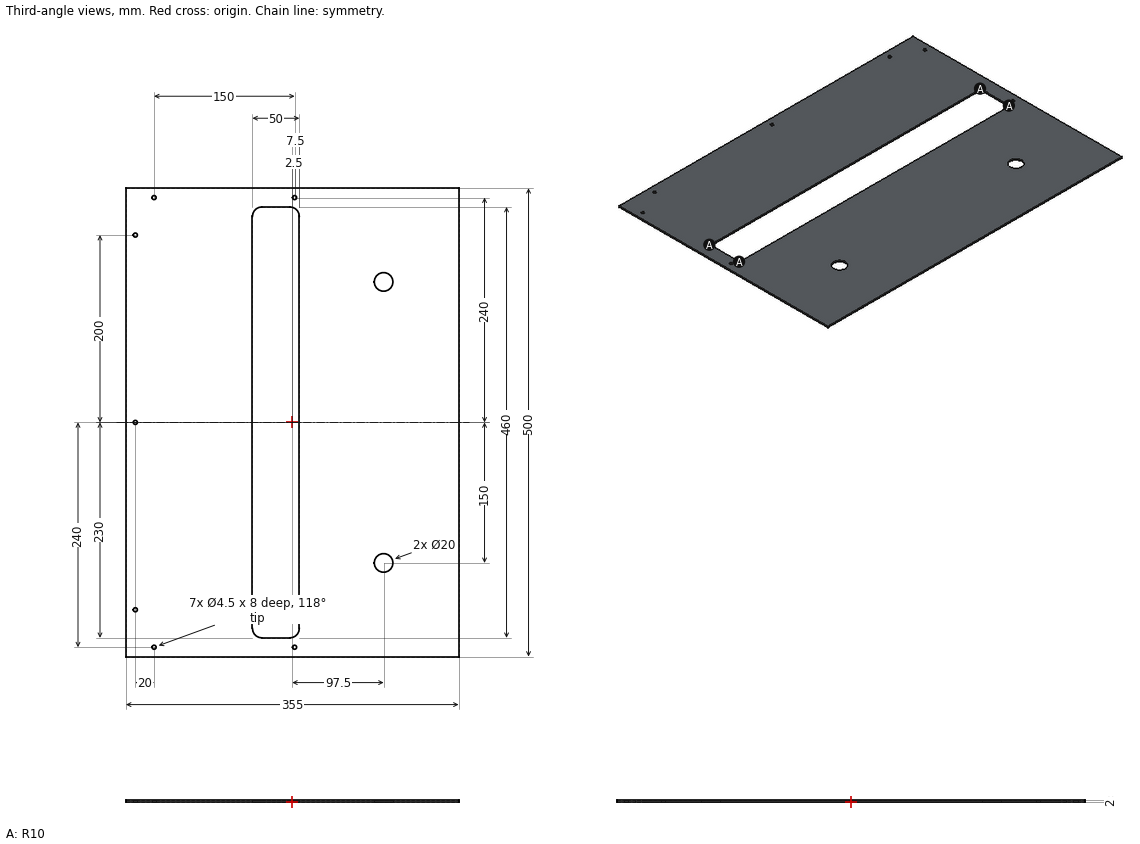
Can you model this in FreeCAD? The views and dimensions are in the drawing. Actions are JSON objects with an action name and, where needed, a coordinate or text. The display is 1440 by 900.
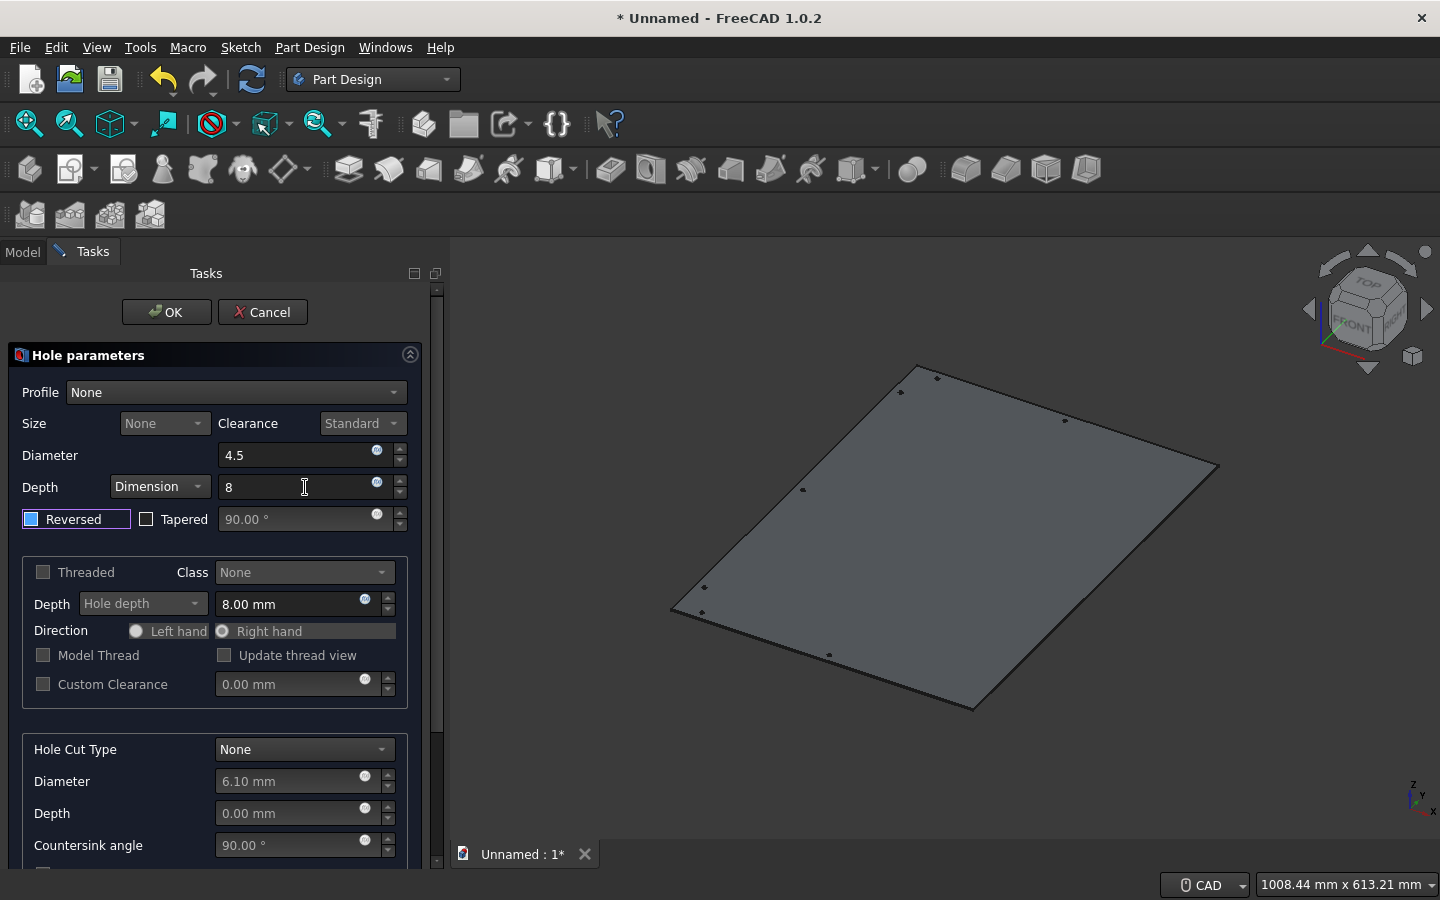
{"action": "left_click", "coordinate": [167, 312]}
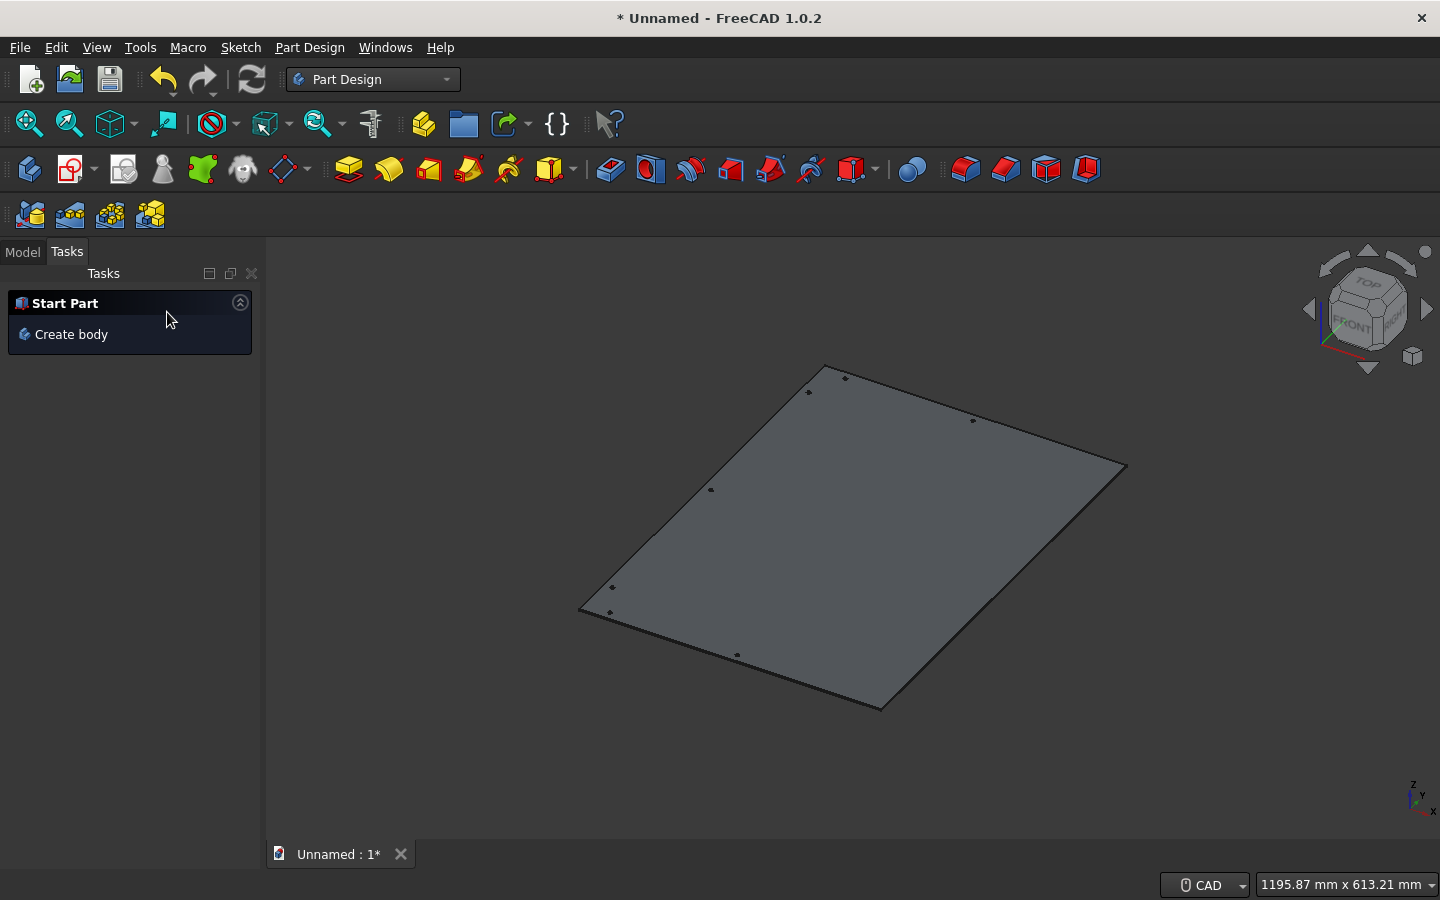
{"action": "key", "text": "5"}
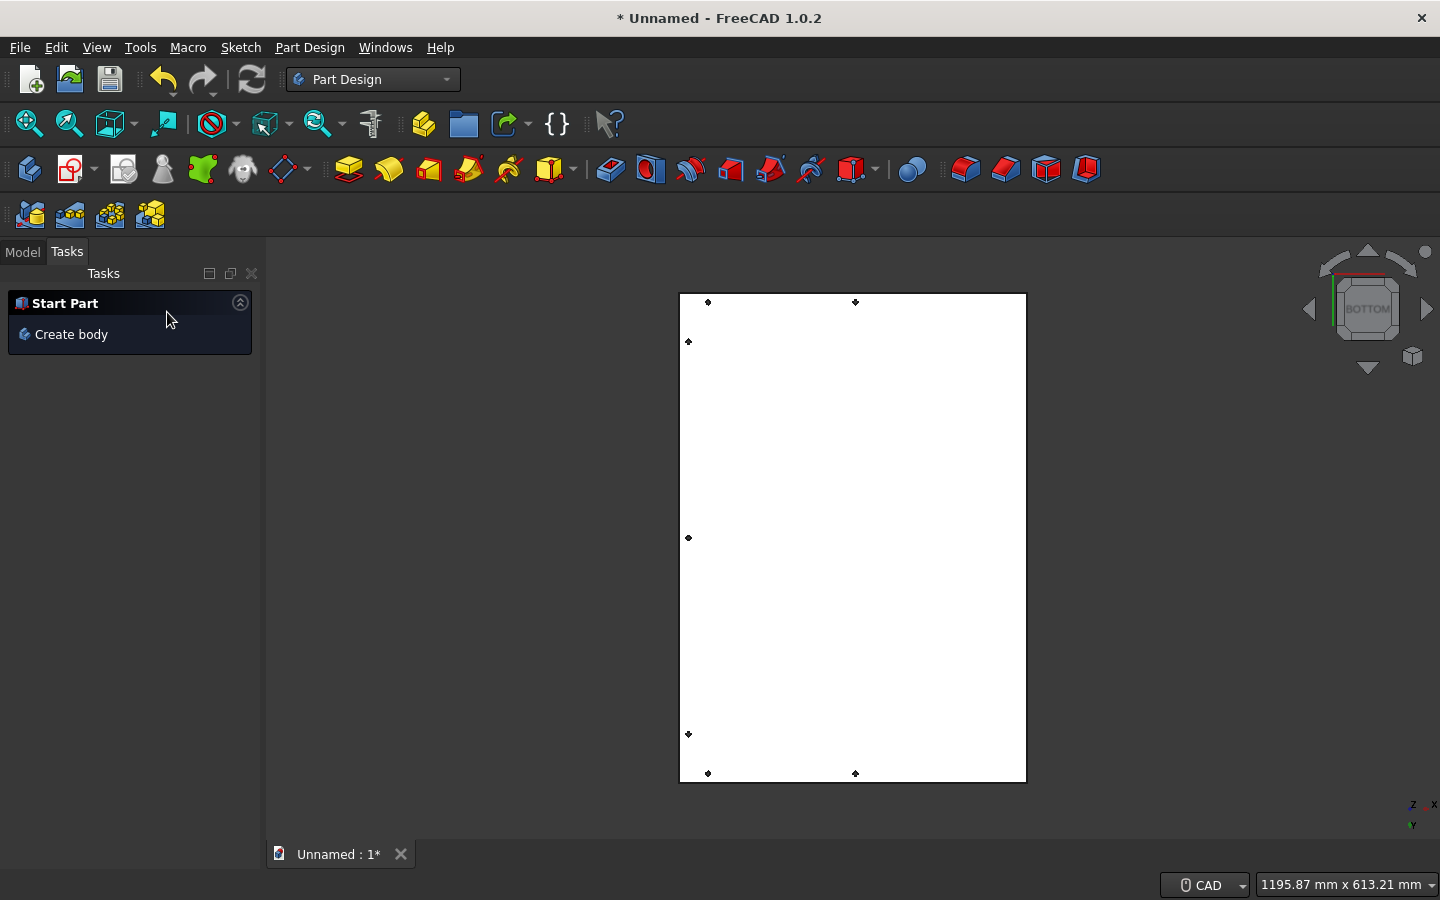
{"action": "left_click", "coordinate": [853, 467]}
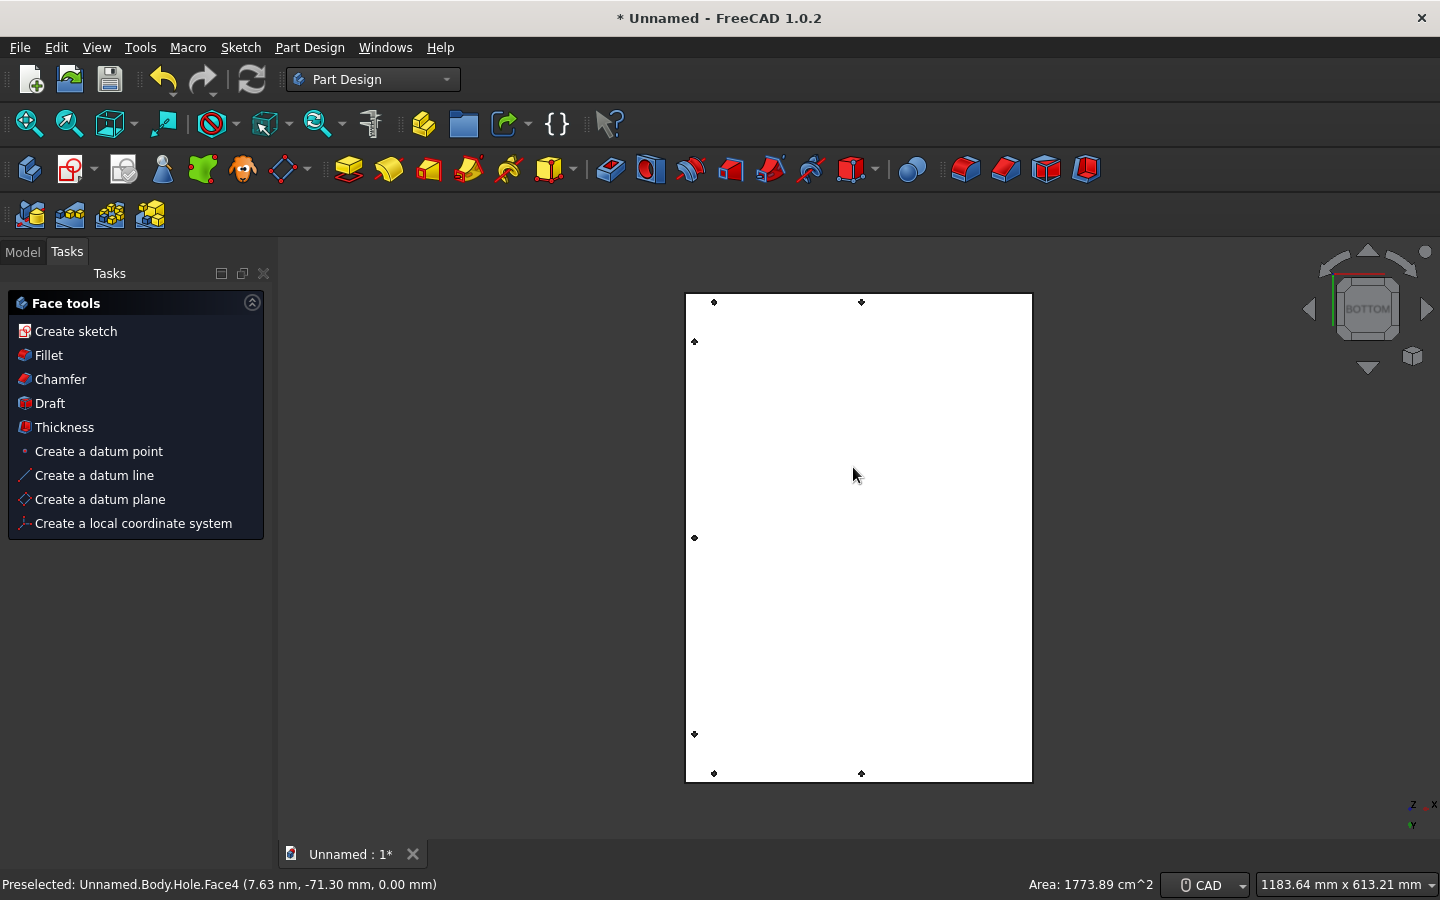
{"action": "left_click", "coordinate": [70, 170]}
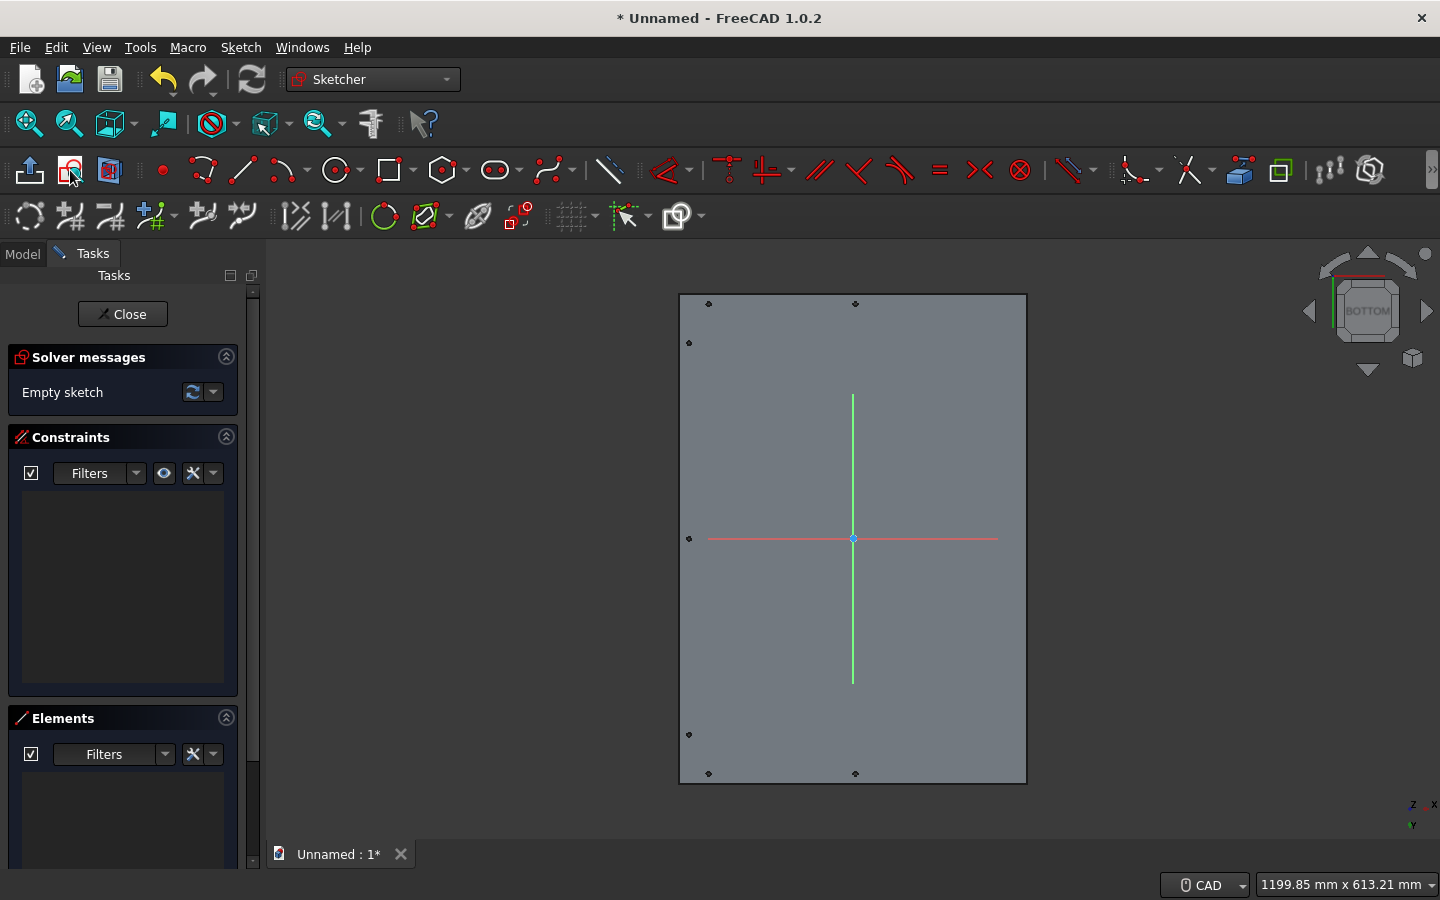
{"action": "left_click", "coordinate": [390, 170]}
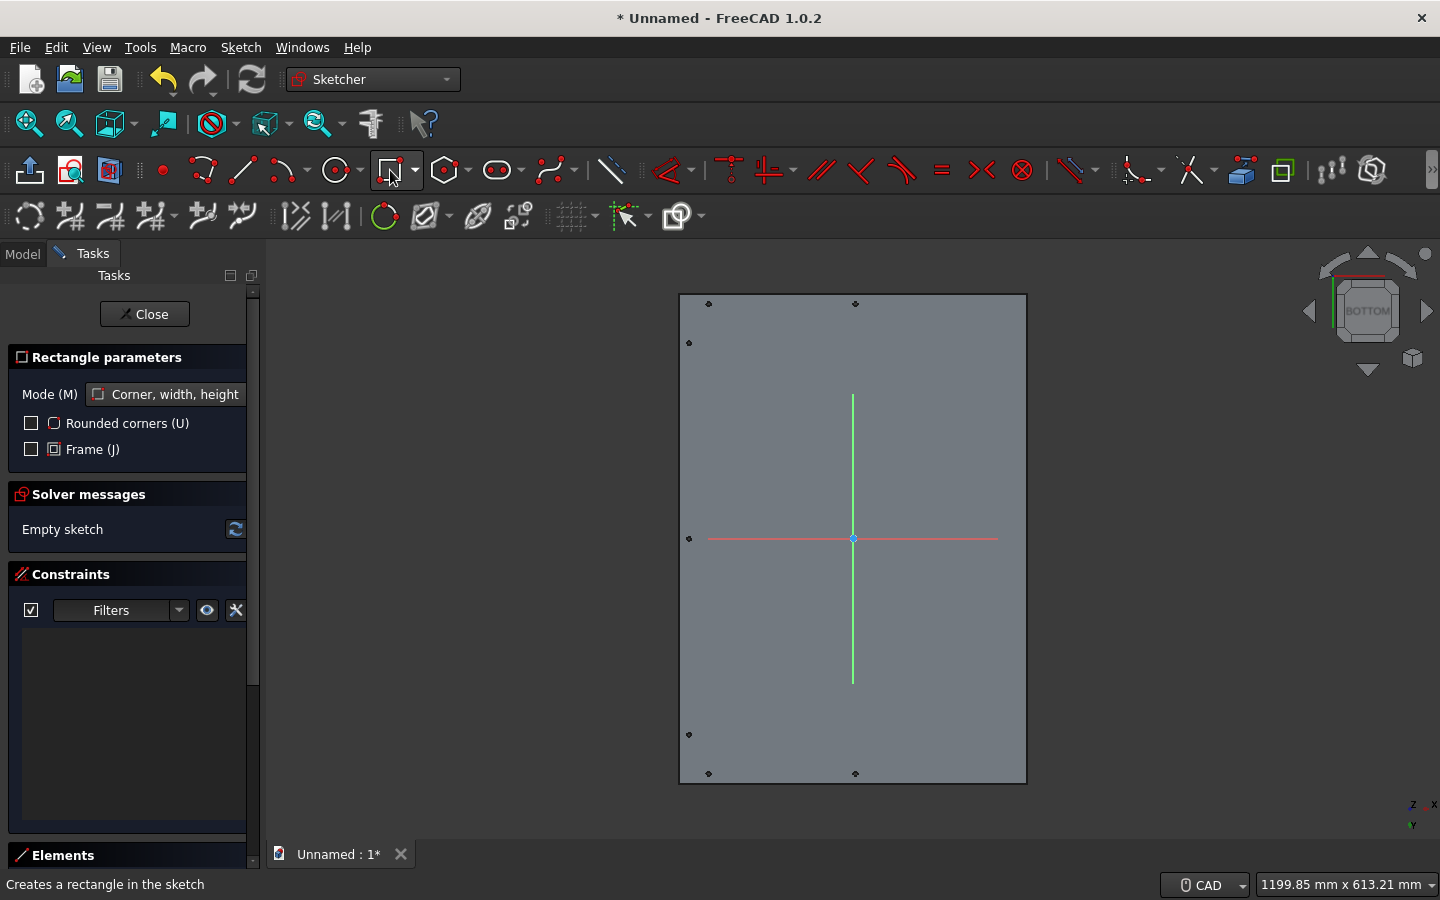
{"action": "left_click", "coordinate": [811, 314]}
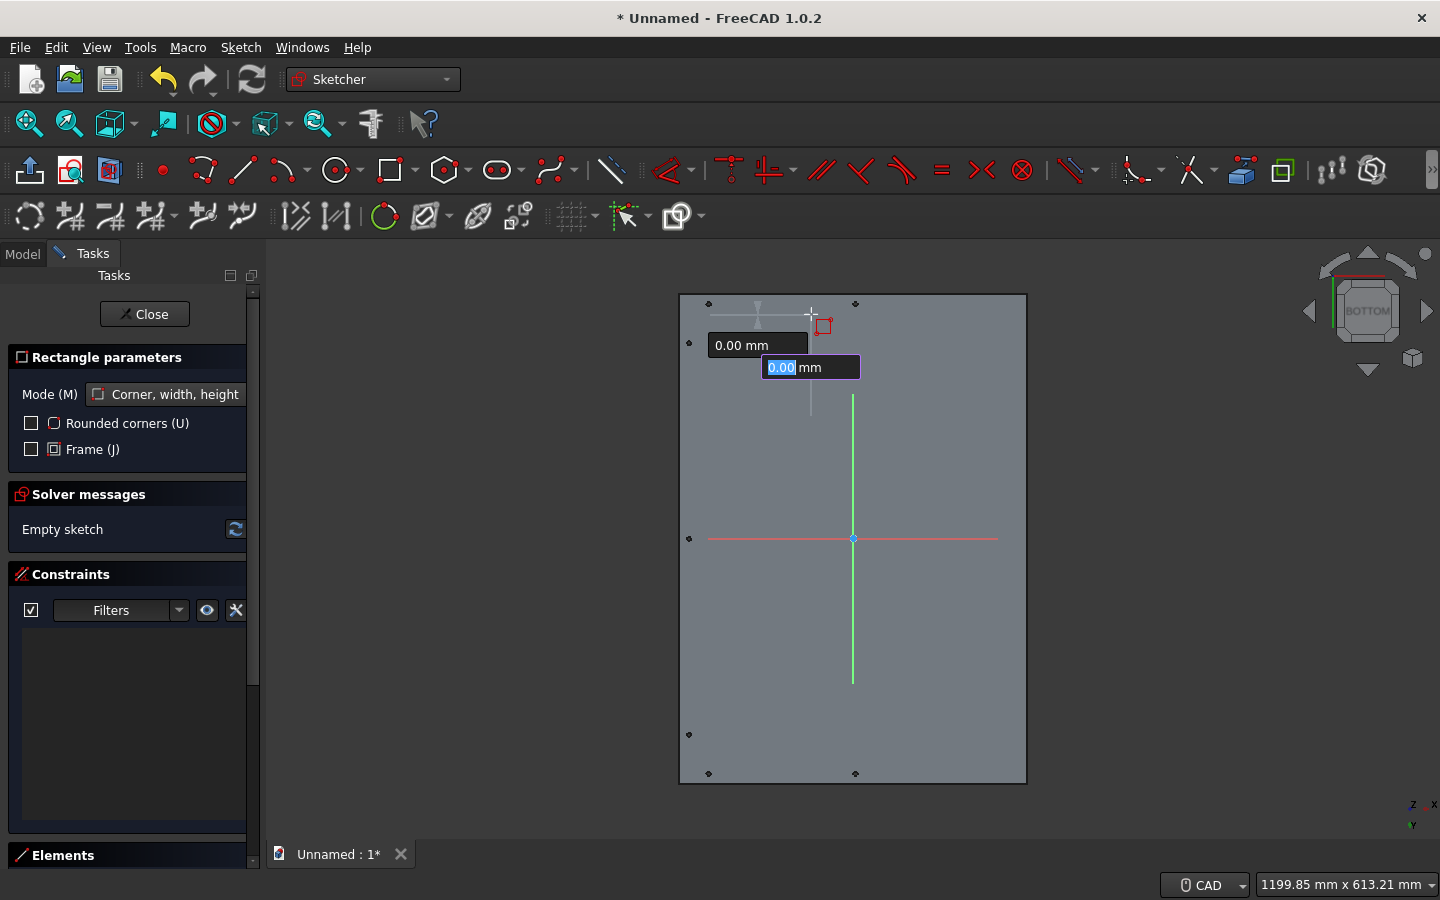
{"action": "scroll", "coordinate": [860, 764], "scroll_direction": "up", "scroll_amount": 4}
{"action": "mouse_move", "coordinate": [860, 763]}